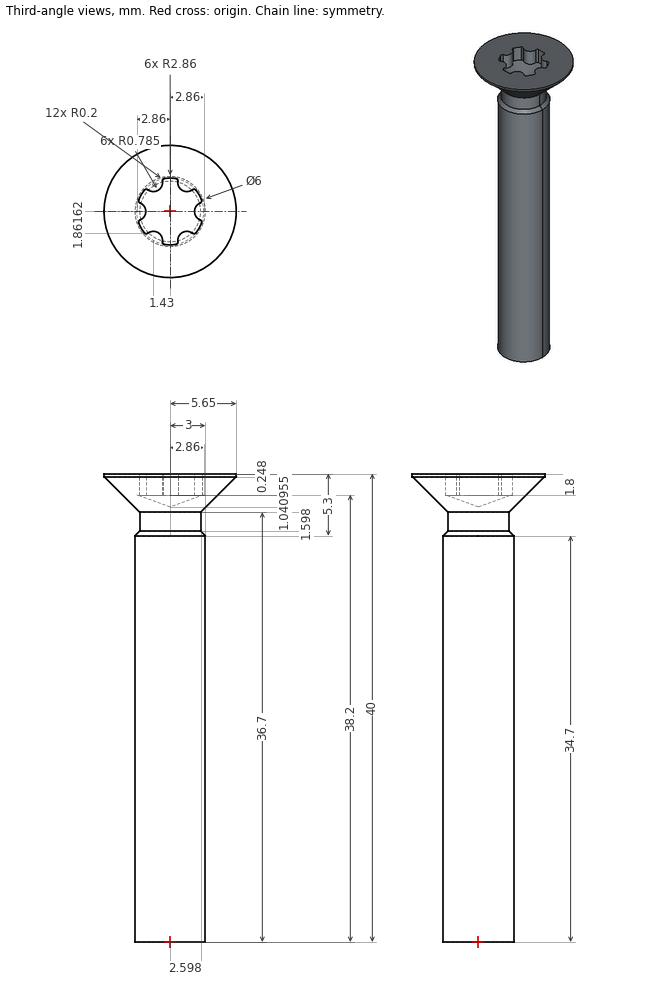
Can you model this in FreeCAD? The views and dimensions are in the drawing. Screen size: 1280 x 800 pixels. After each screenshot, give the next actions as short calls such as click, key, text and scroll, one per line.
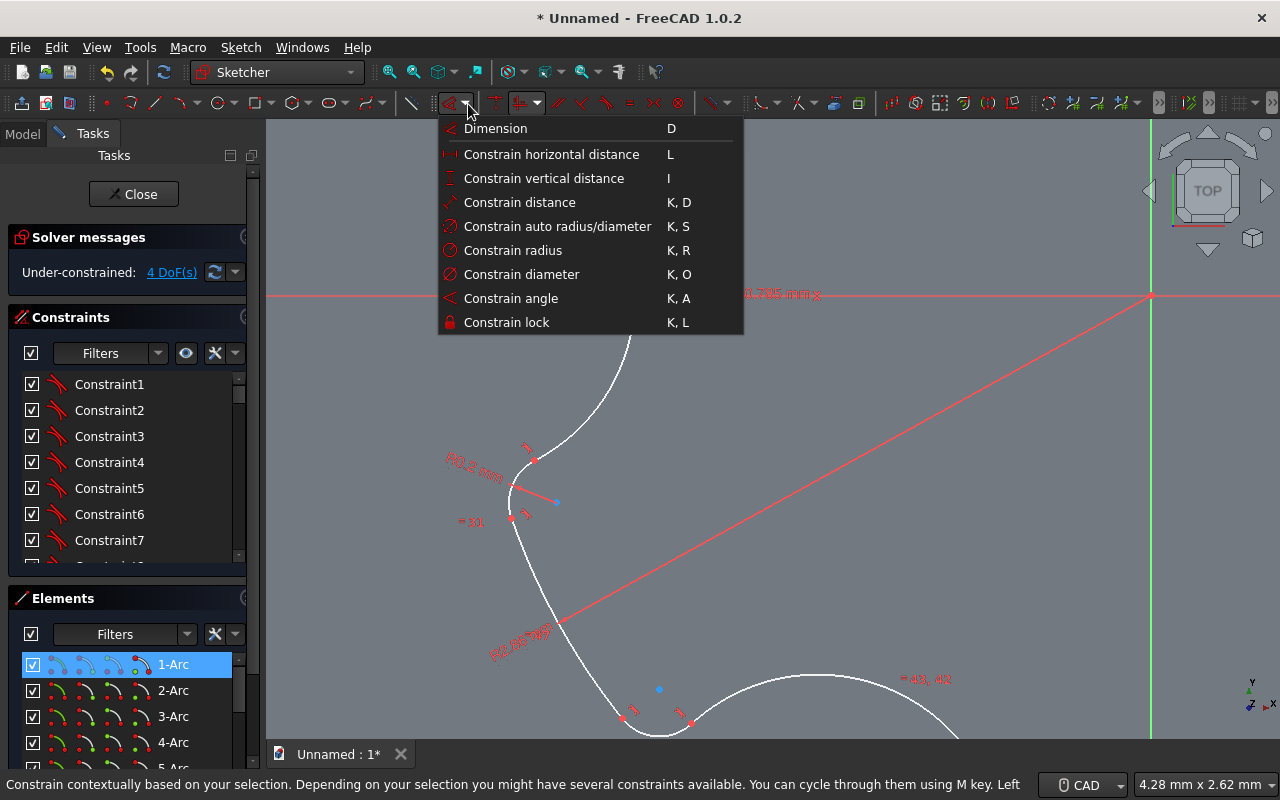
click(591, 154)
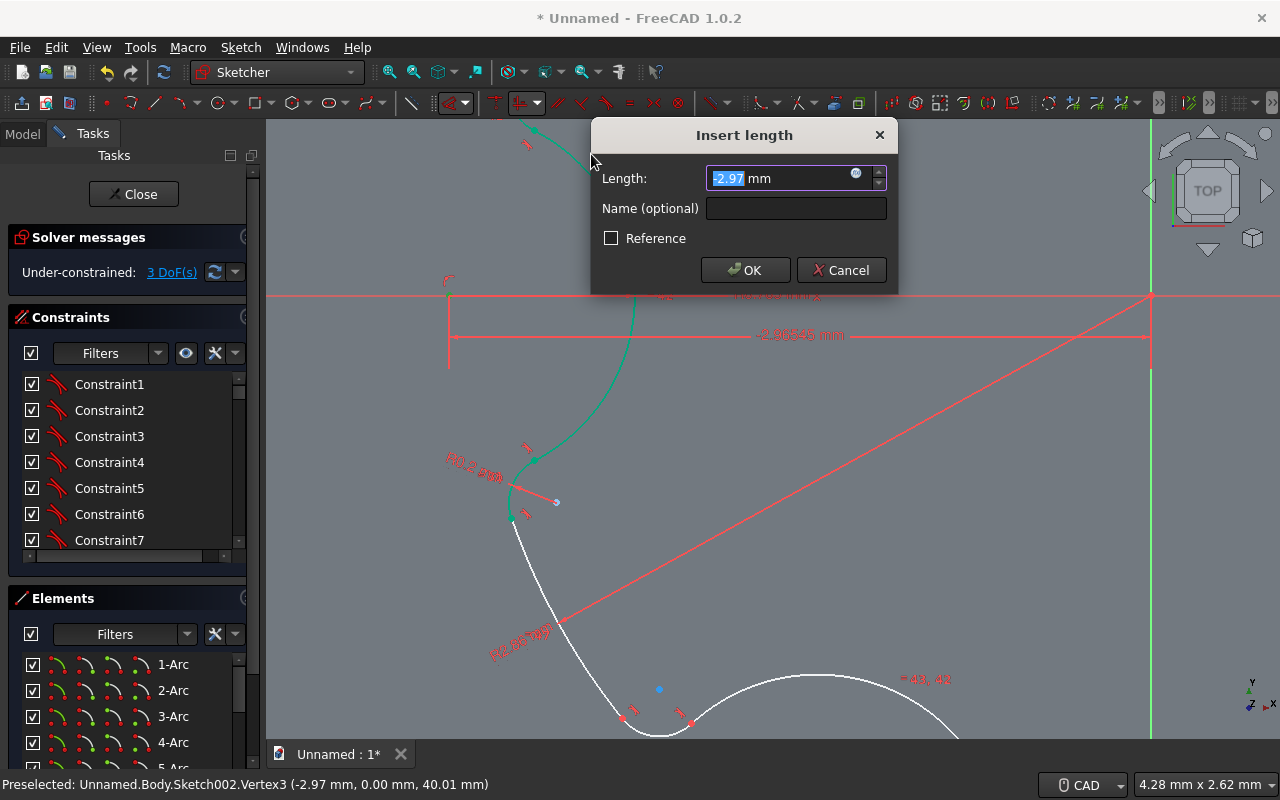
text(-2.86)
key(Return)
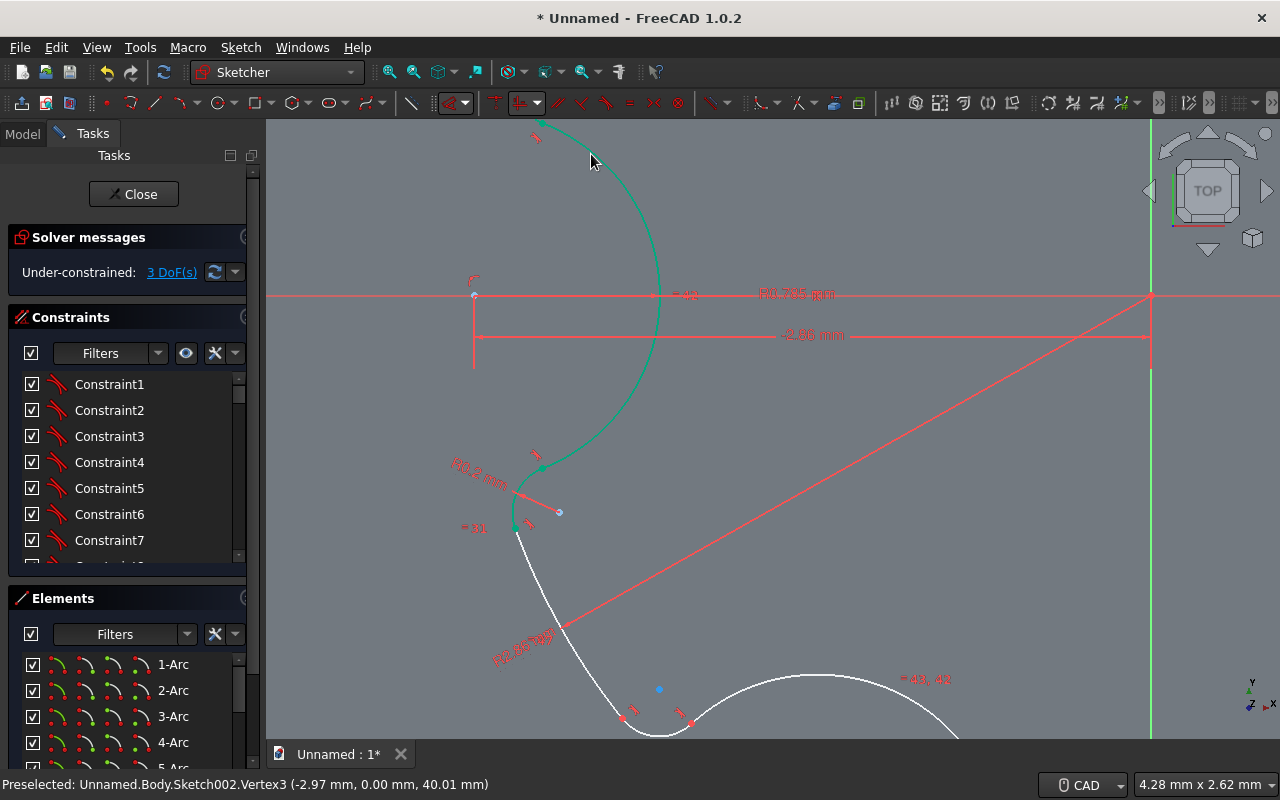
scroll(512, 486, down, 6)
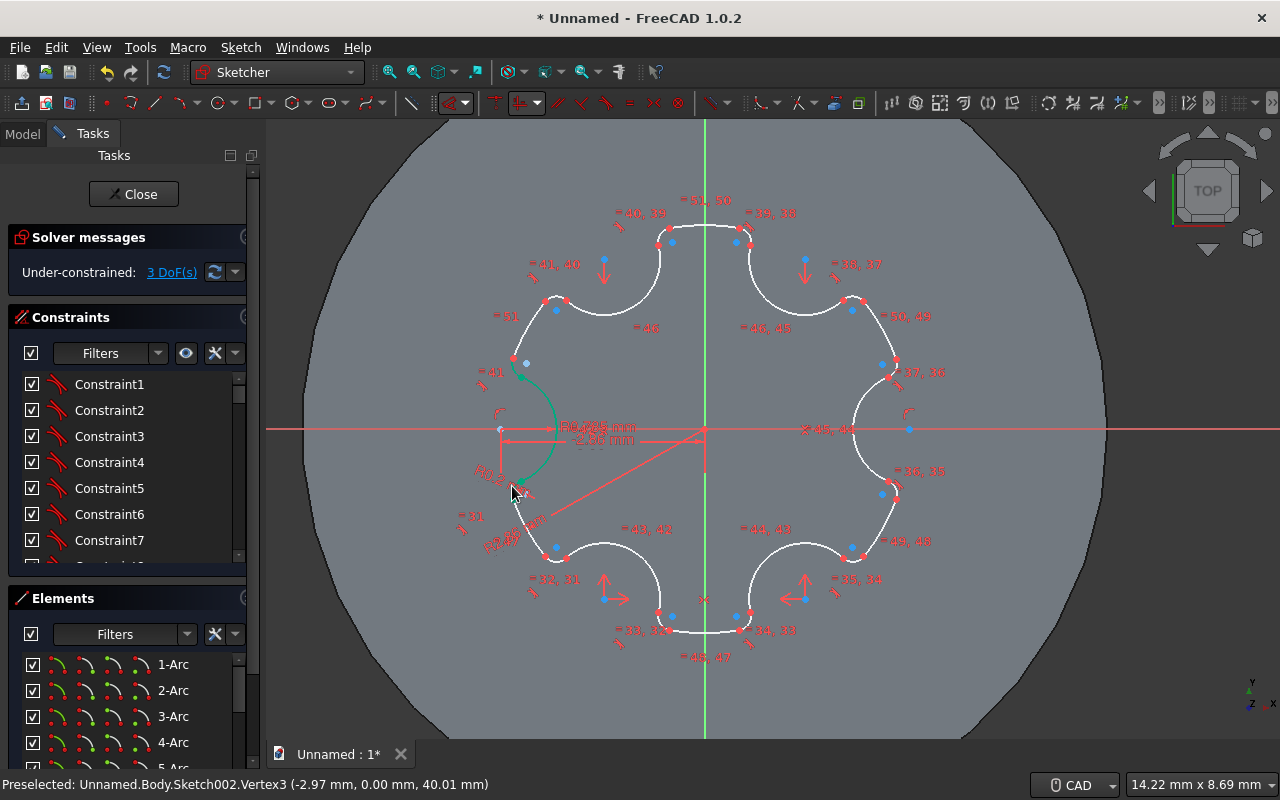
click(604, 599)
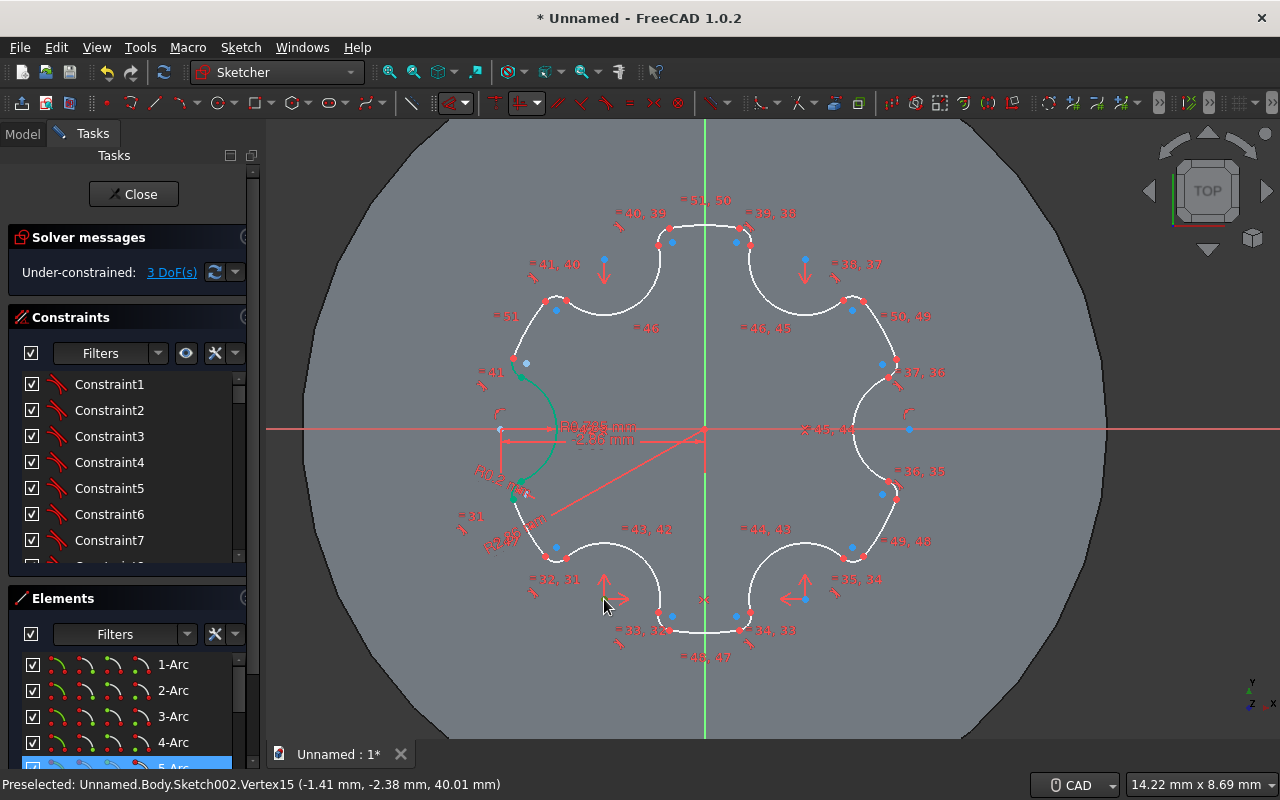
key(l)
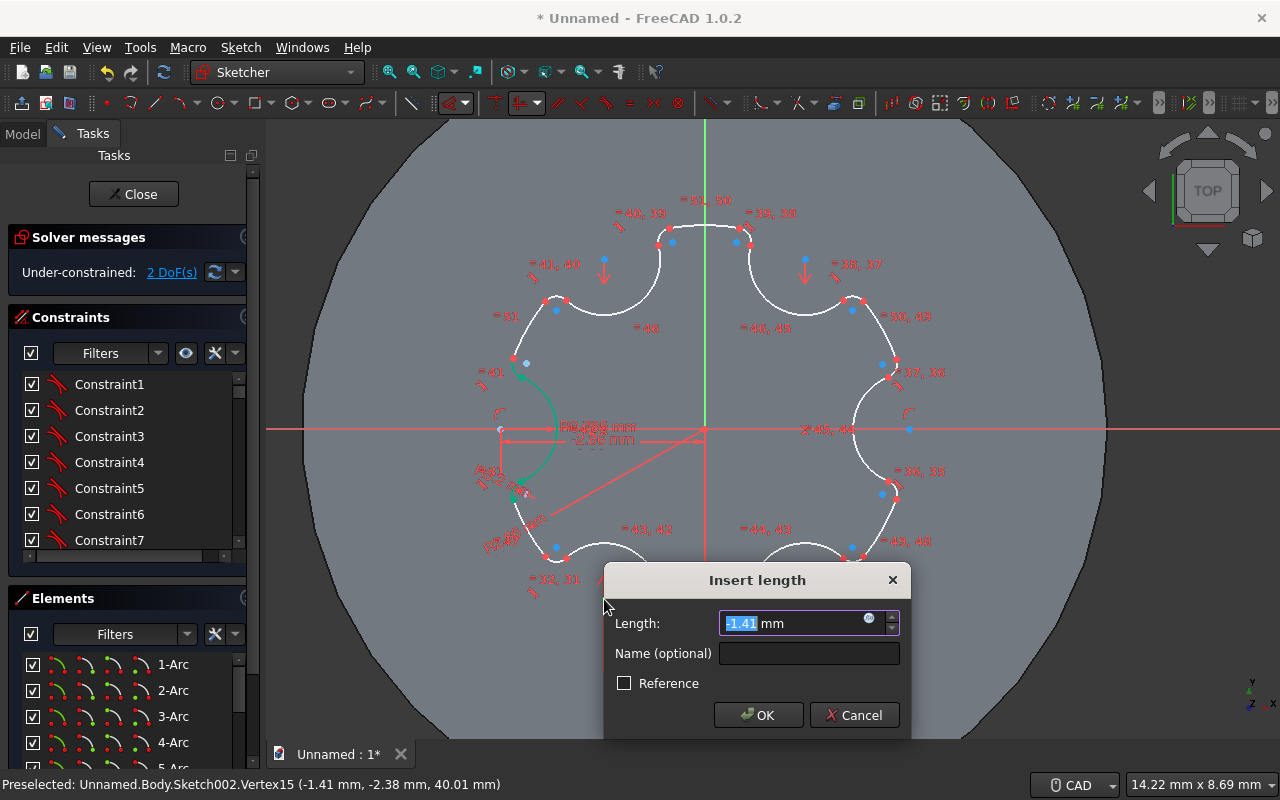
text(-1.43)
key(Return)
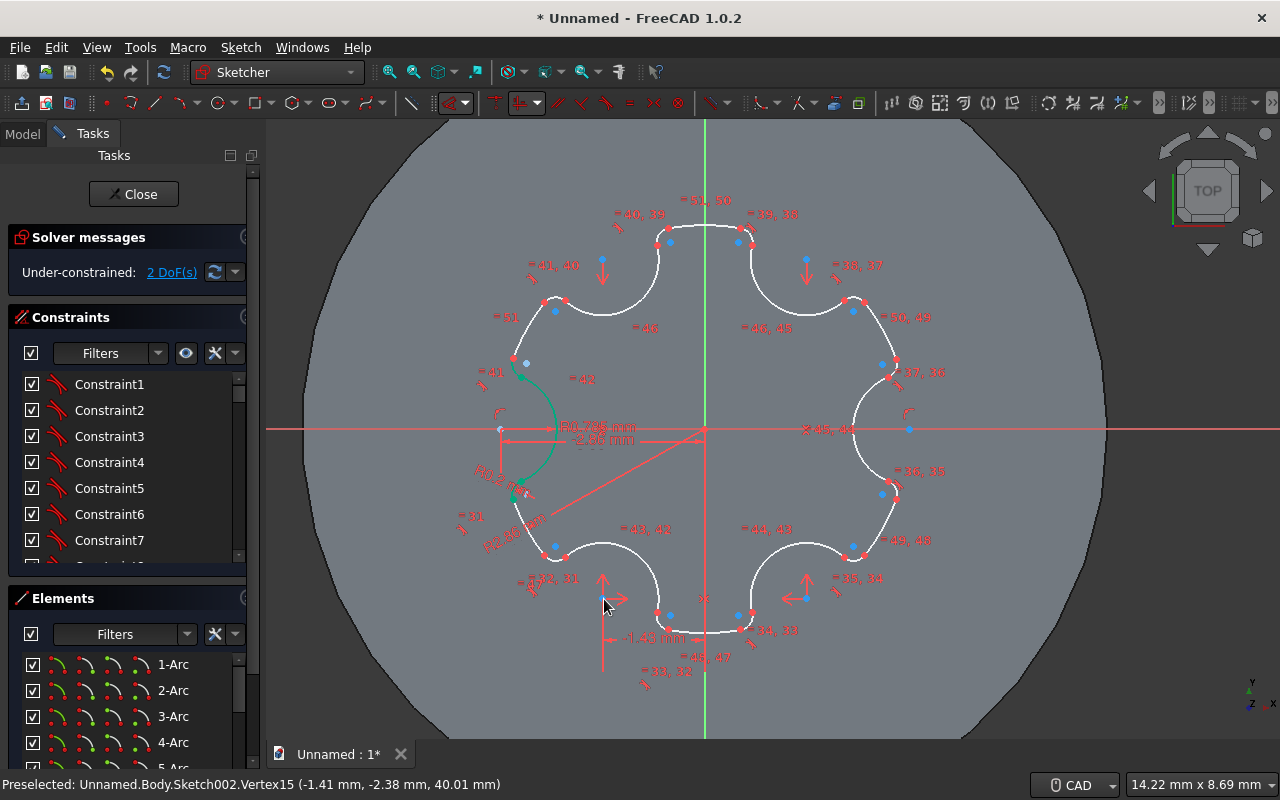
click(909, 429)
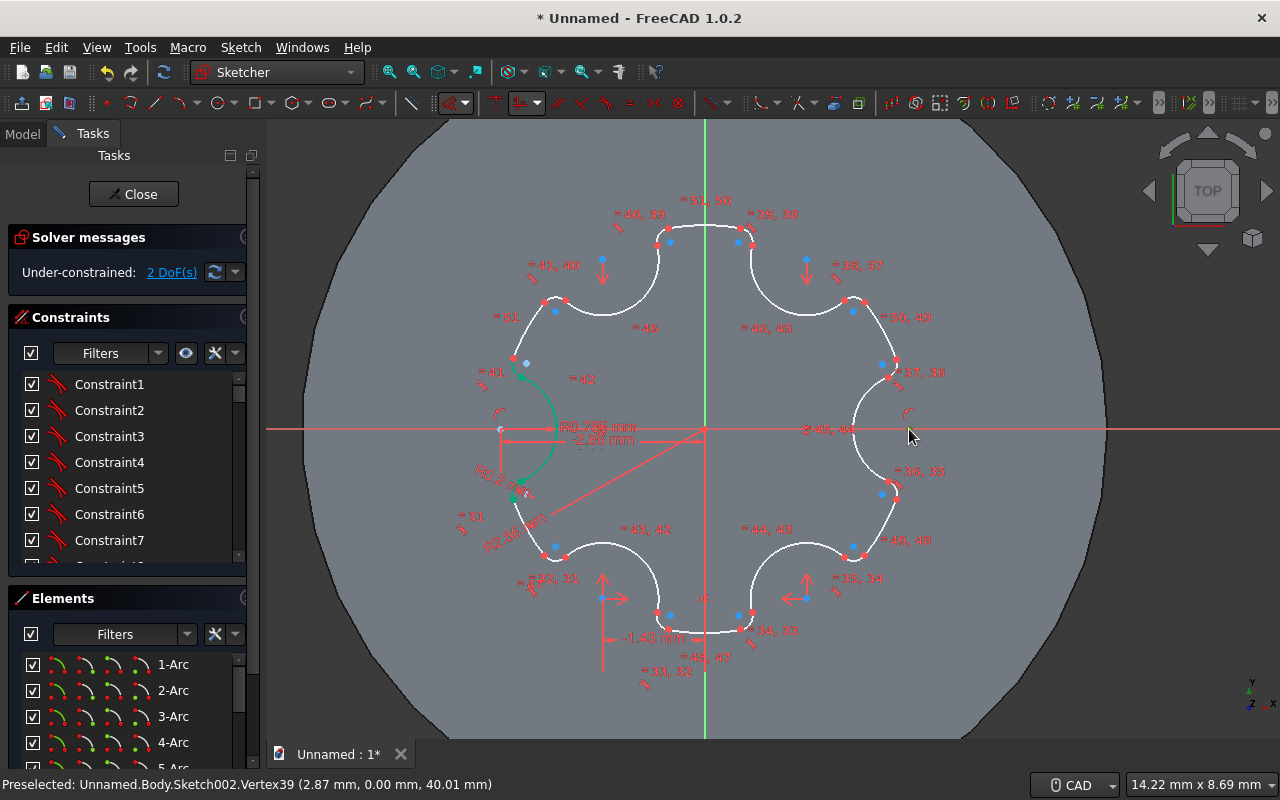
key(l)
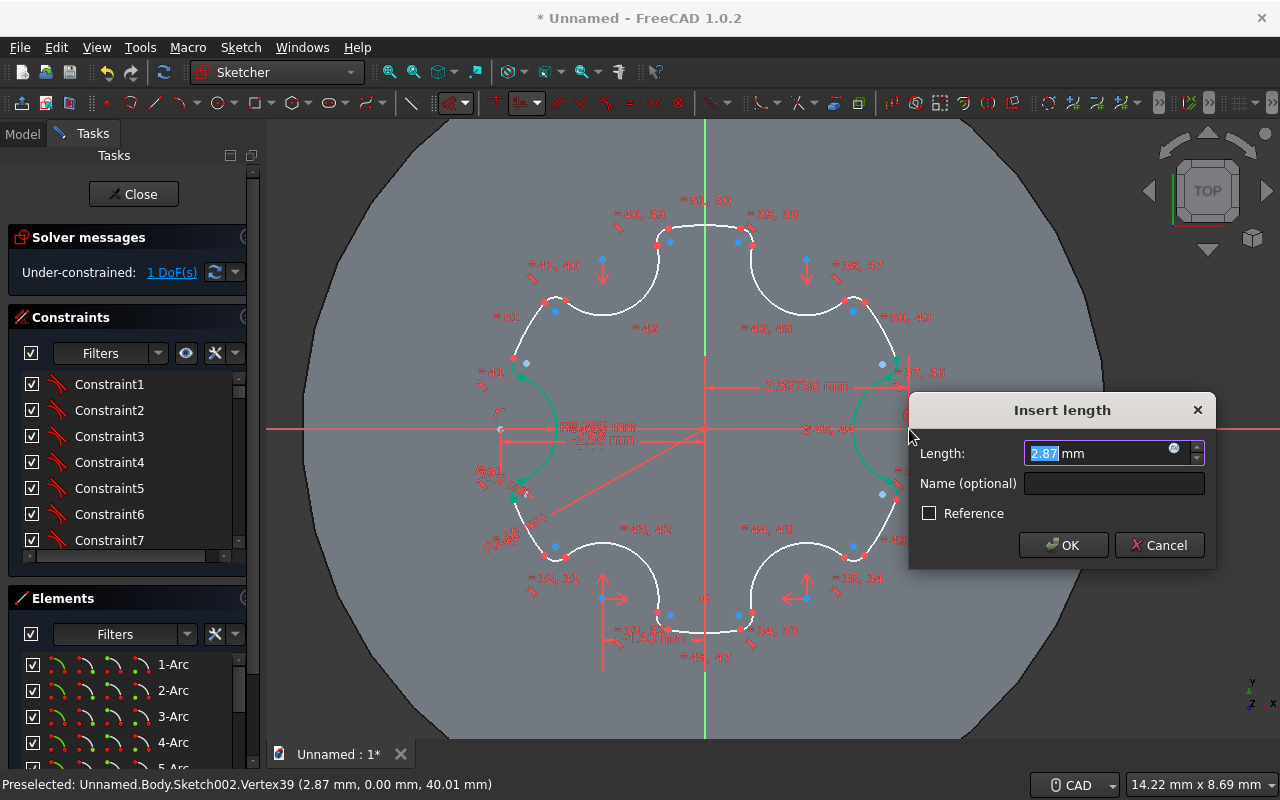
text(2.86)
key(Return)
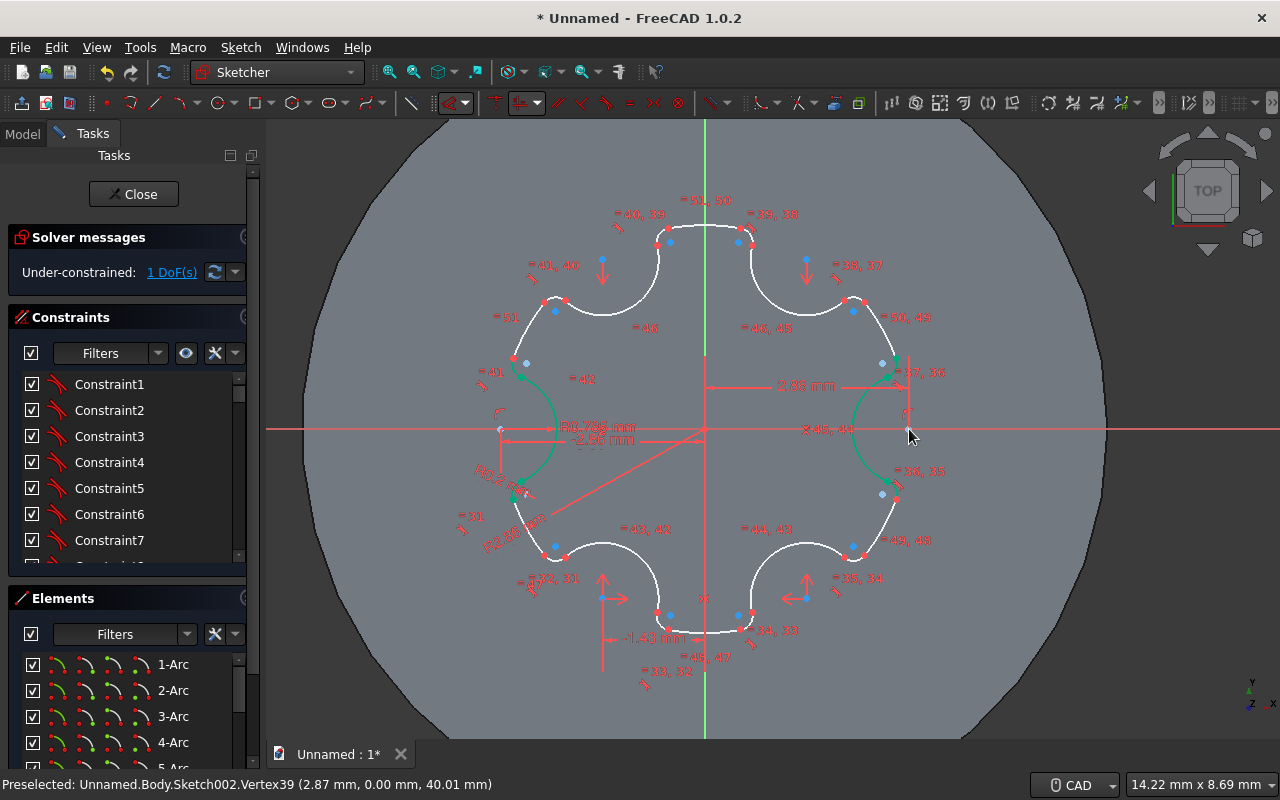
click(565, 557)